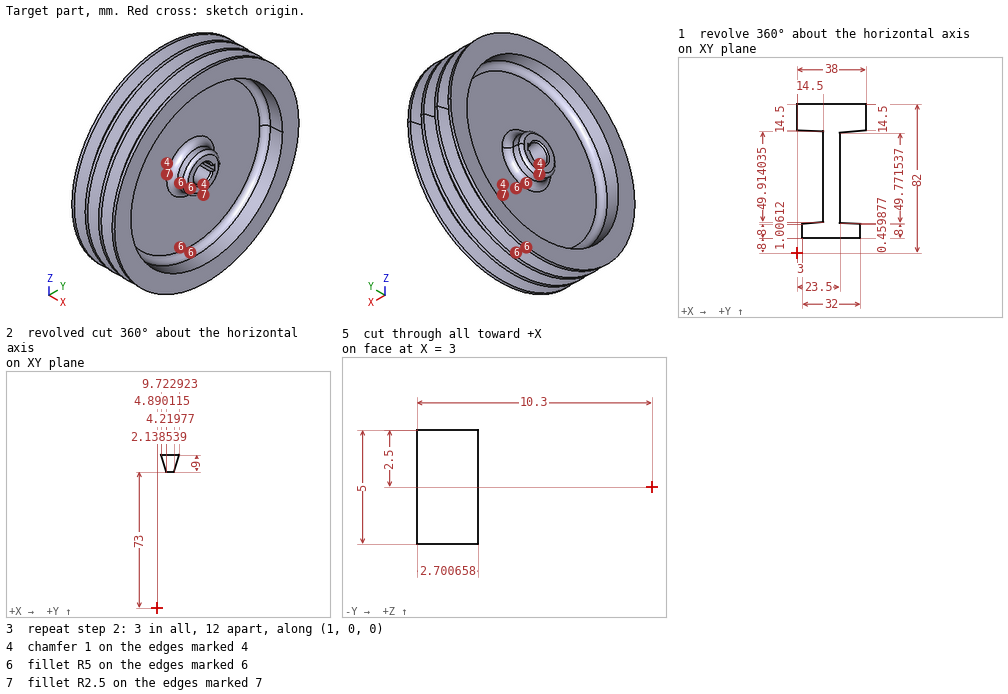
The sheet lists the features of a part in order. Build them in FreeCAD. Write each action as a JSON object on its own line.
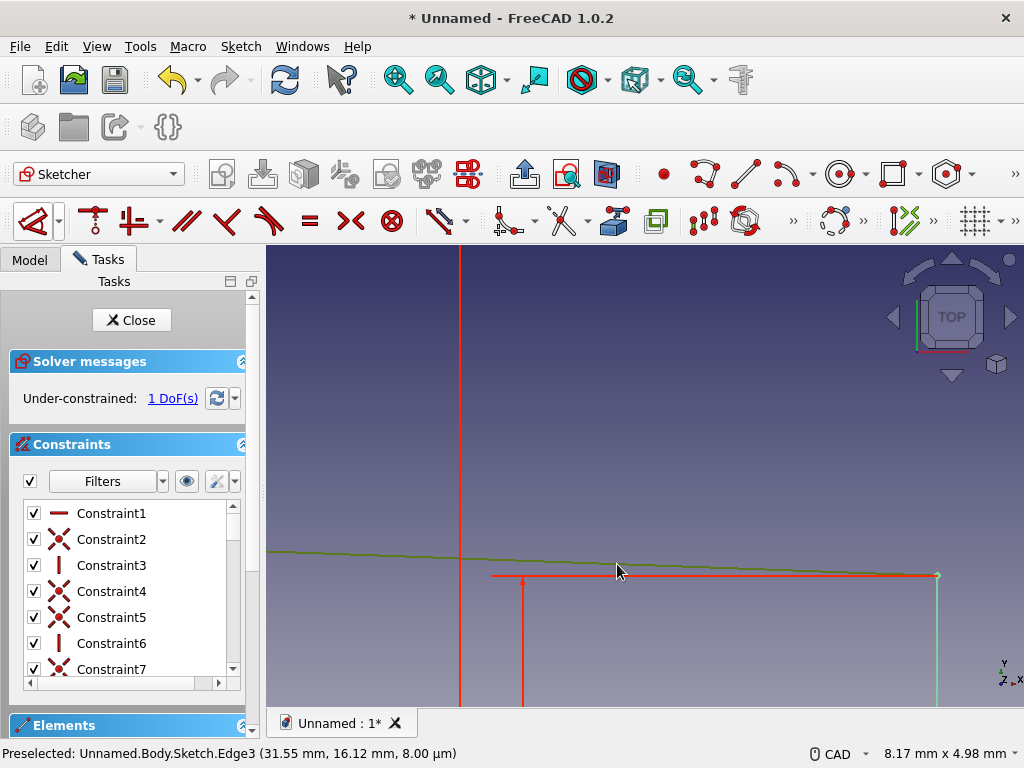
{"action": "key", "text": "i"}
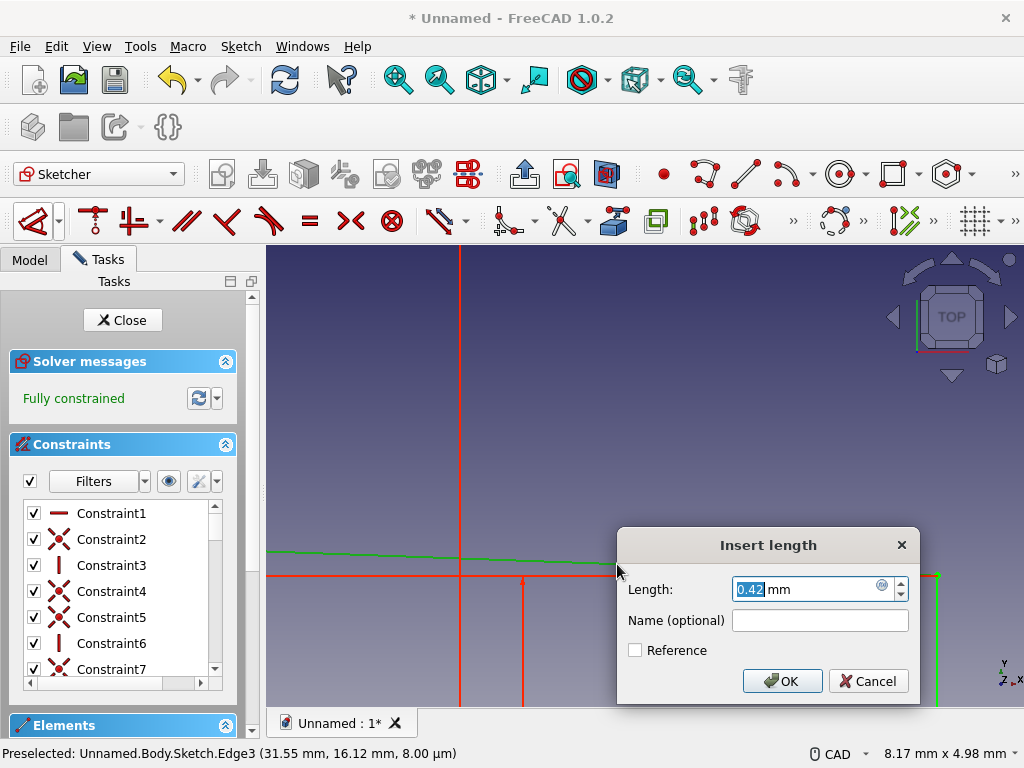
{"action": "type", "text": "0.459877"}
{"action": "key", "text": "Return"}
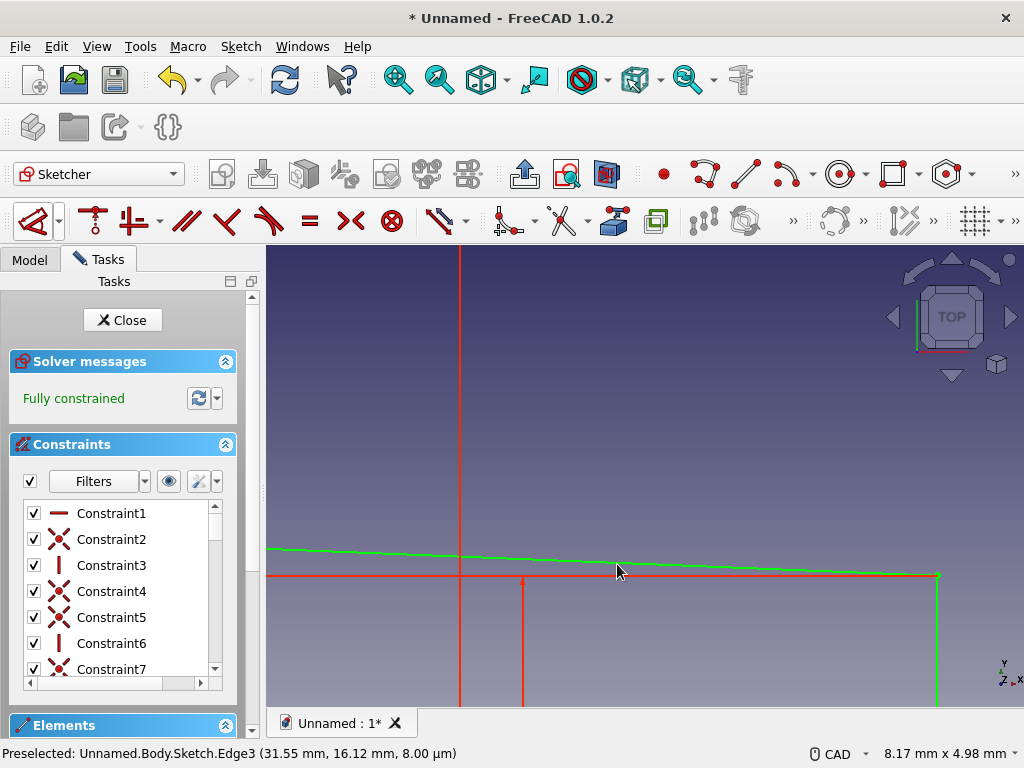
{"action": "left_click", "coordinate": [123, 320]}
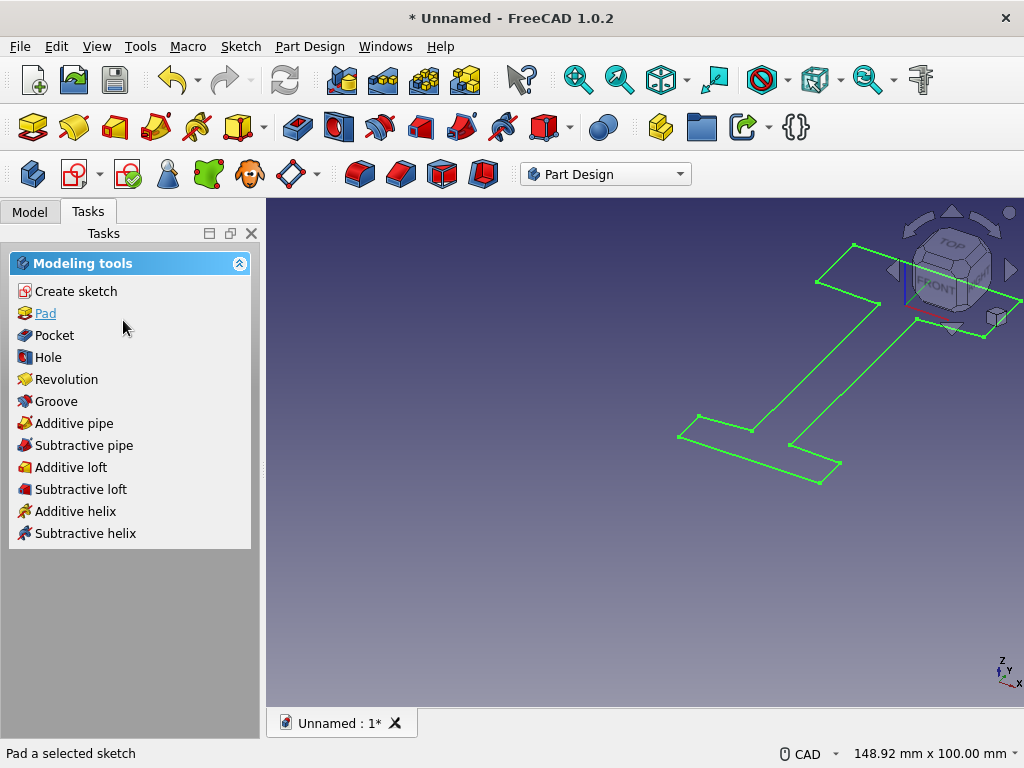
{"action": "left_click", "coordinate": [74, 128]}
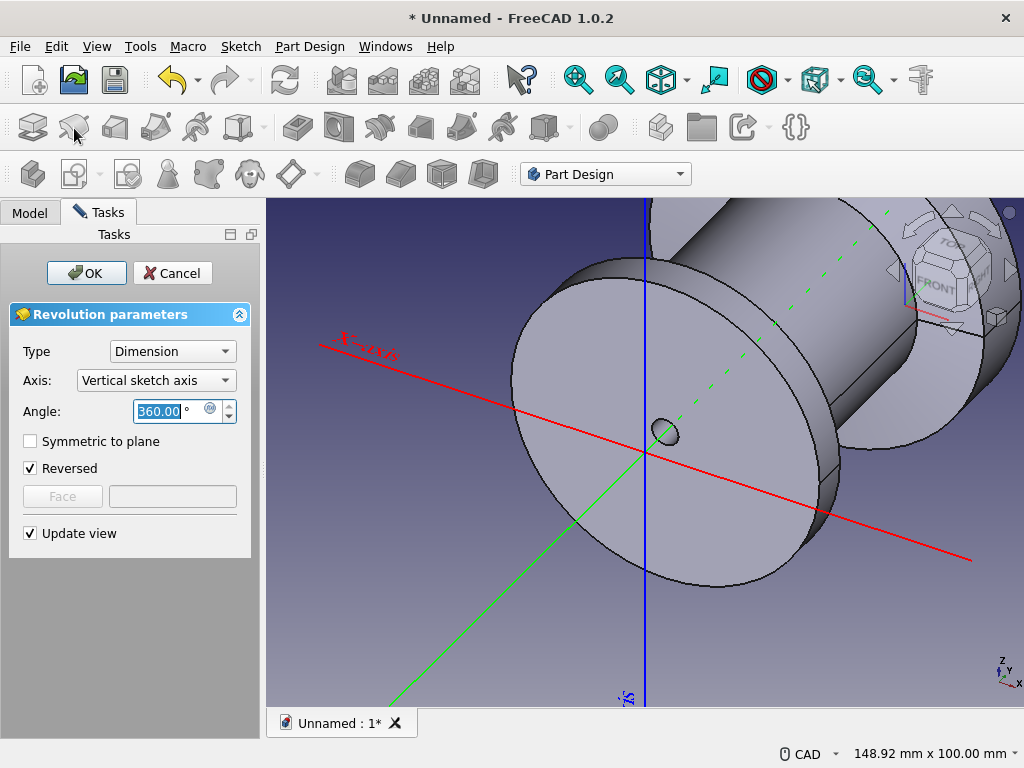
{"action": "left_click", "coordinate": [157, 380]}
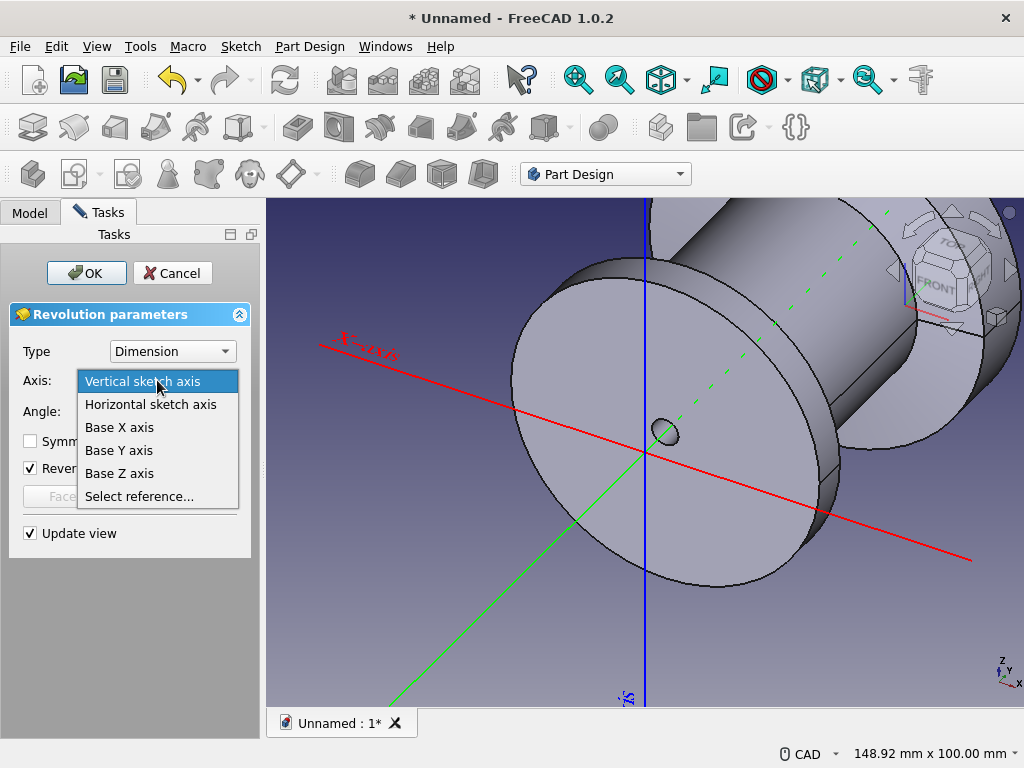
{"action": "left_click", "coordinate": [156, 404]}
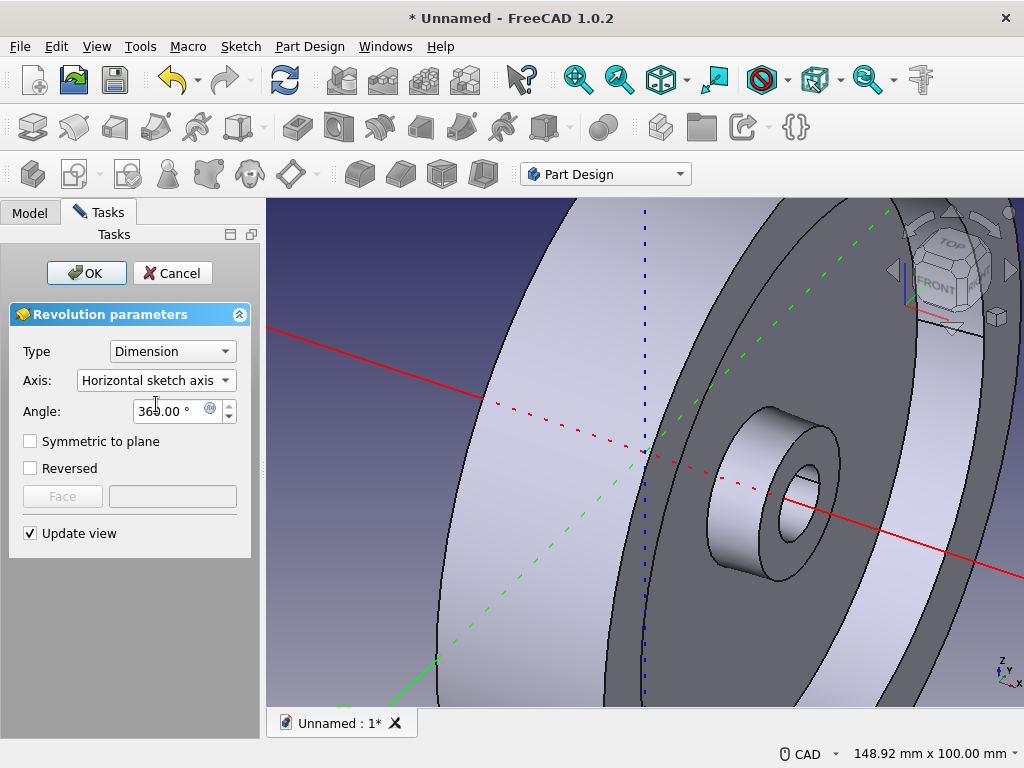
{"action": "left_click", "coordinate": [87, 273]}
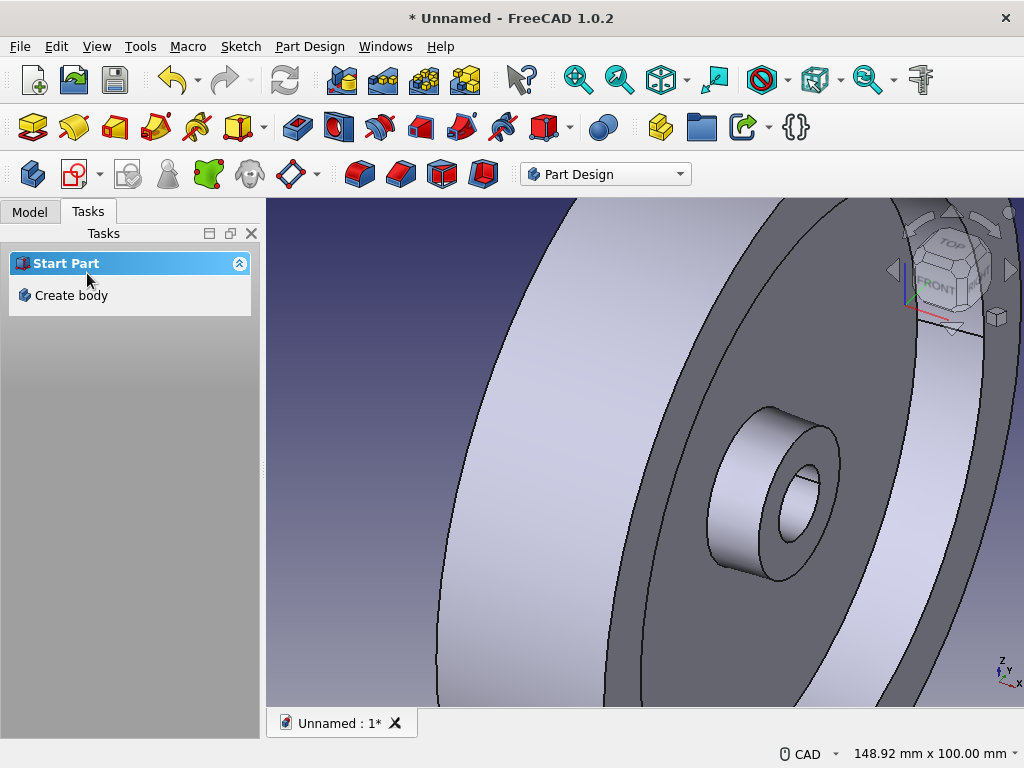
{"action": "left_click", "coordinate": [579, 80]}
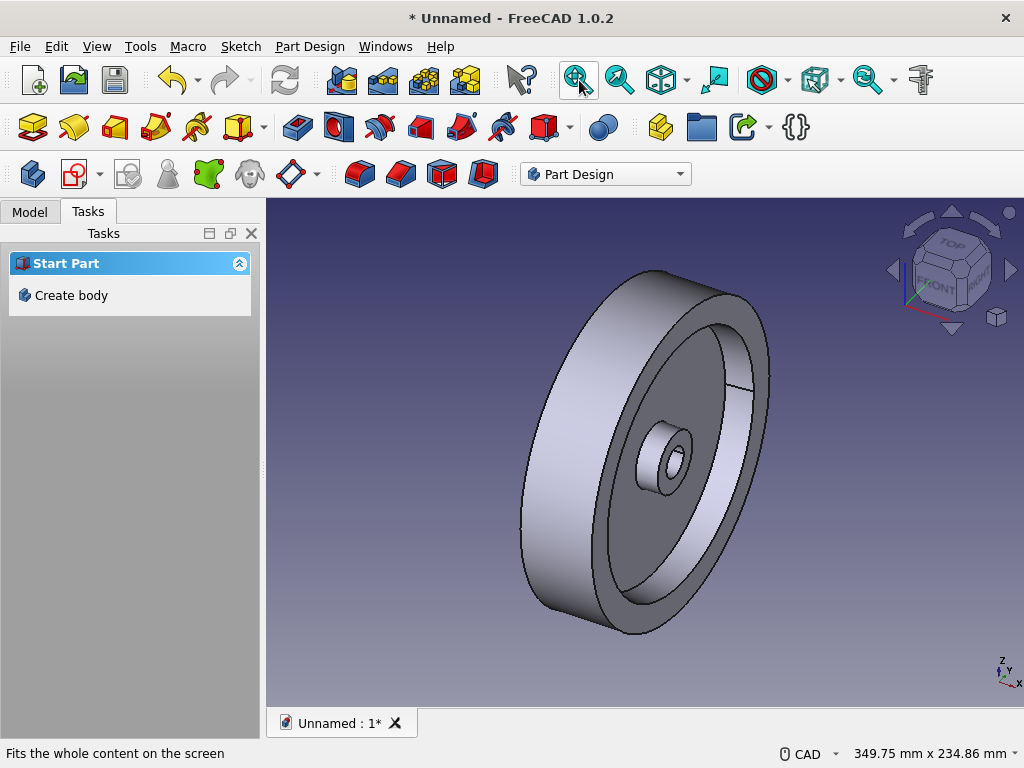
{"action": "left_click", "coordinate": [74, 174]}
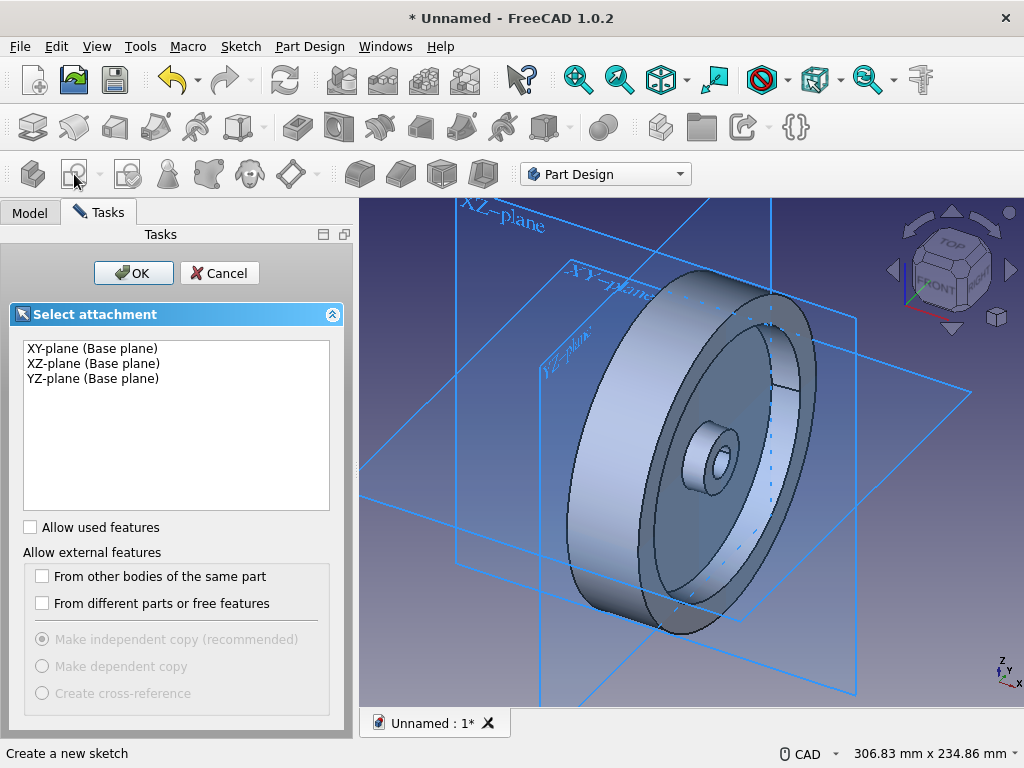
{"action": "left_click", "coordinate": [84, 348]}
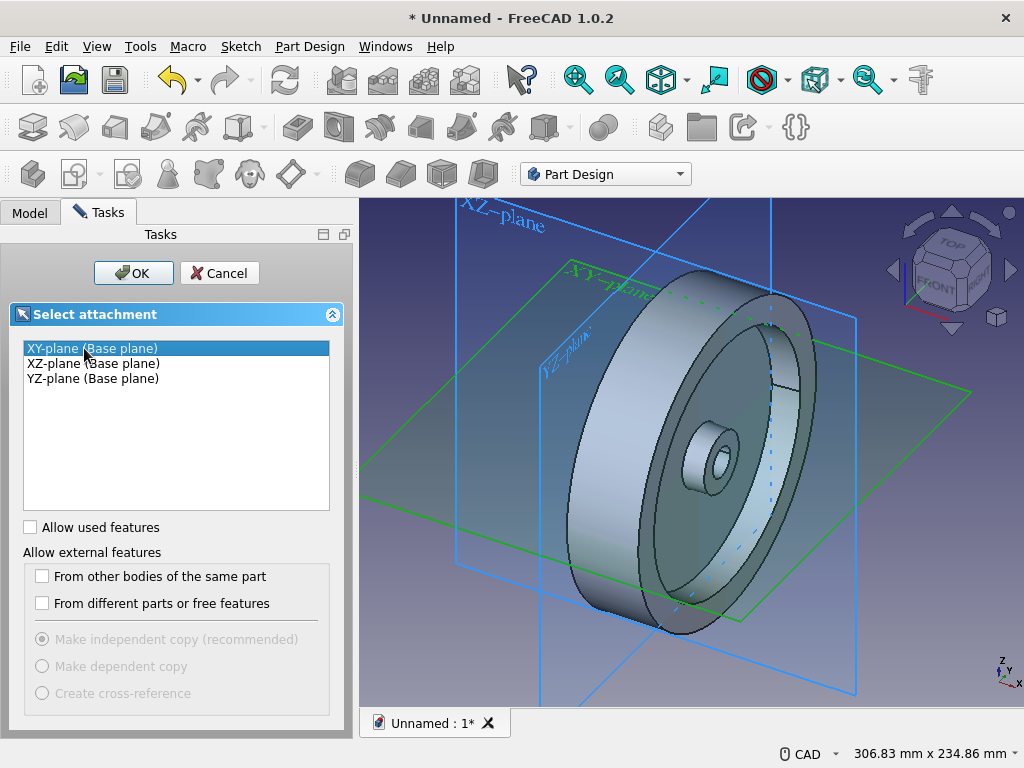
{"action": "left_click", "coordinate": [134, 273]}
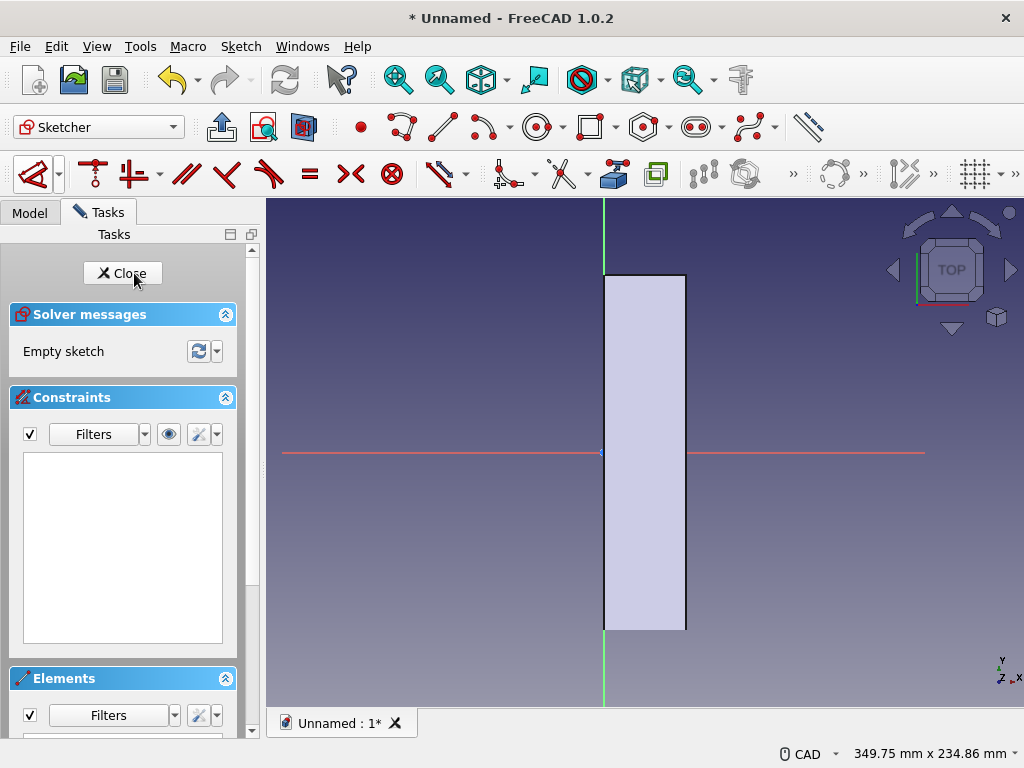
{"action": "left_click", "coordinate": [304, 128]}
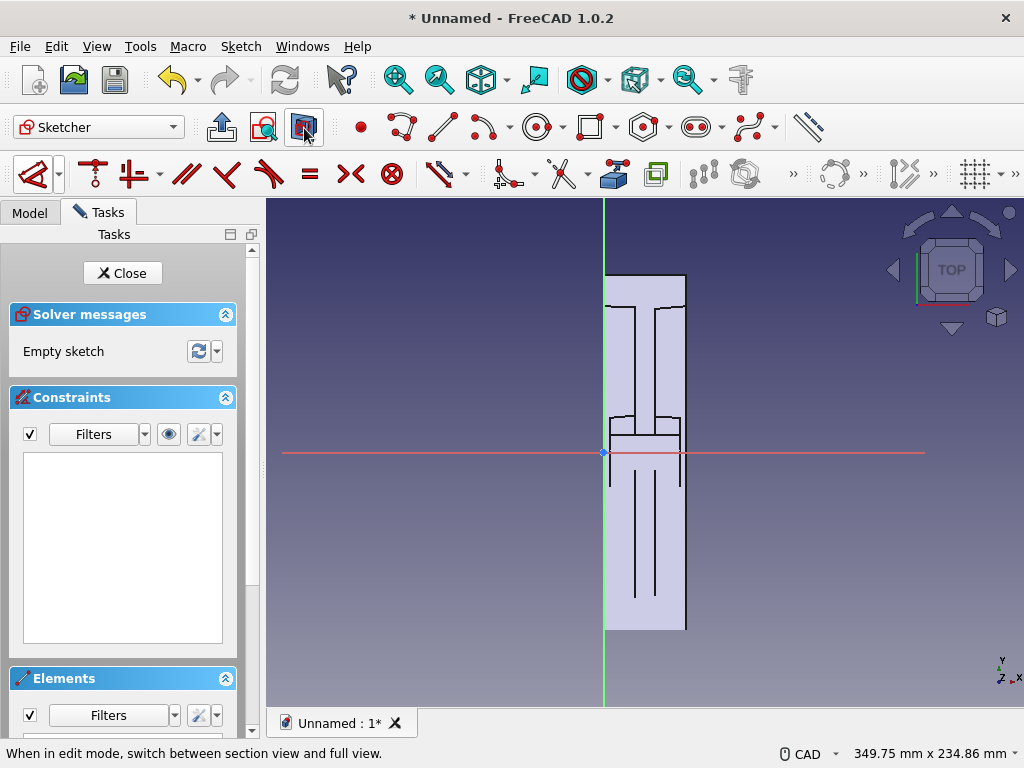
{"action": "scroll", "coordinate": [622, 274], "scroll_direction": "up", "scroll_amount": 14}